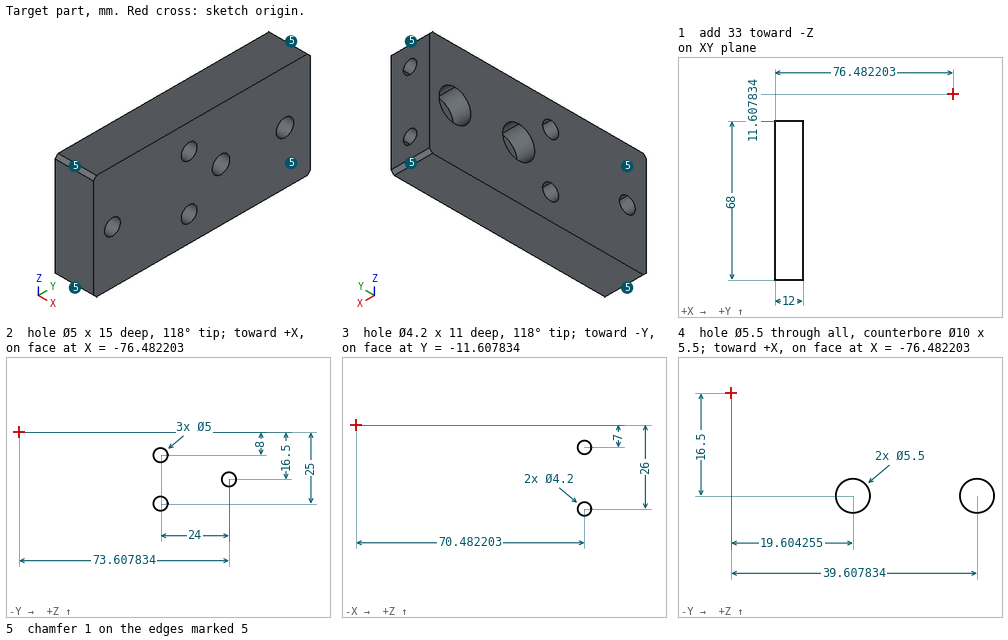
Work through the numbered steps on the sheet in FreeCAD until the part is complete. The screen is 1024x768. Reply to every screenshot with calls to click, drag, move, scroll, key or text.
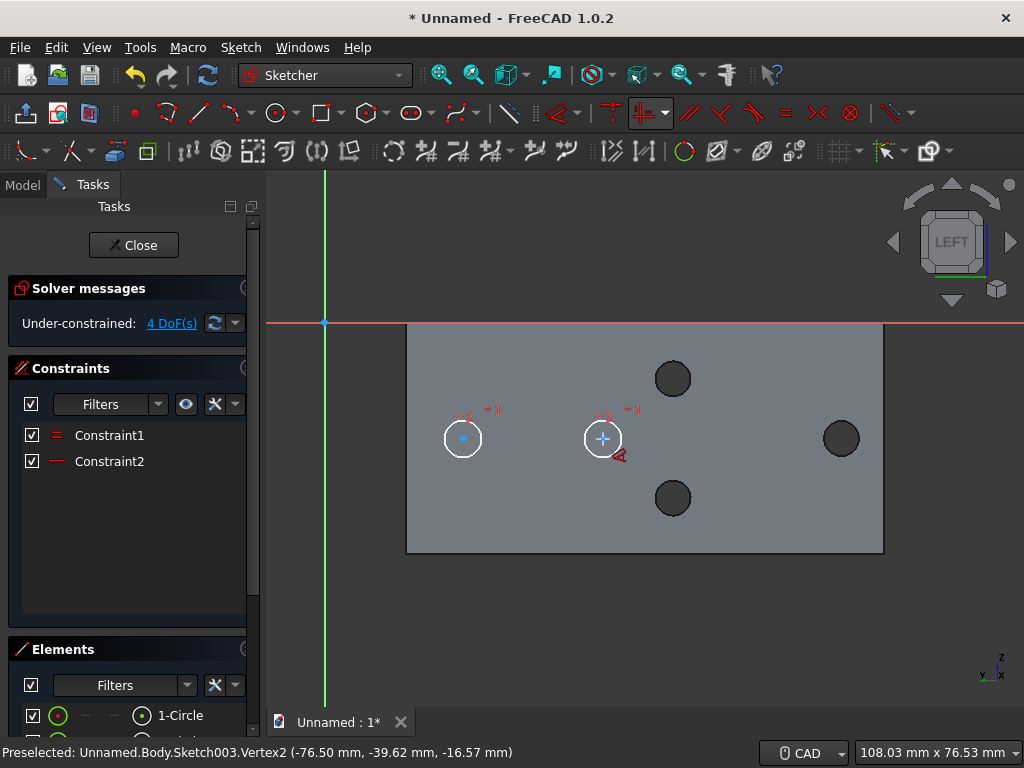
click(476, 426)
click(499, 403)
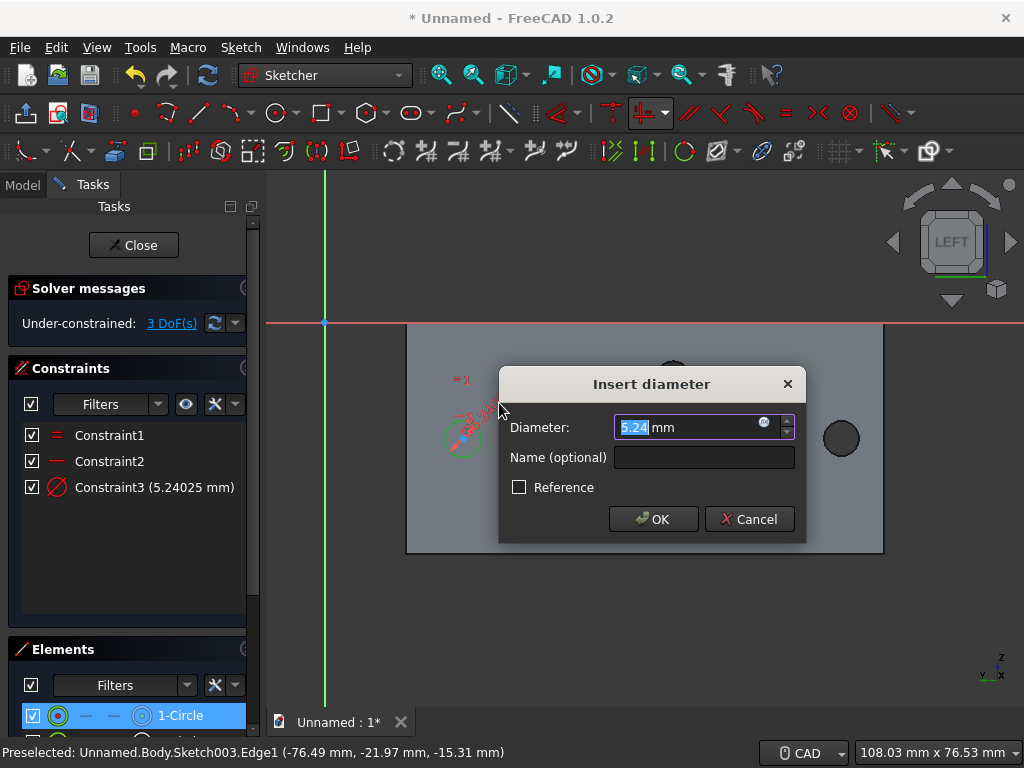
text(5.5)
key(Return)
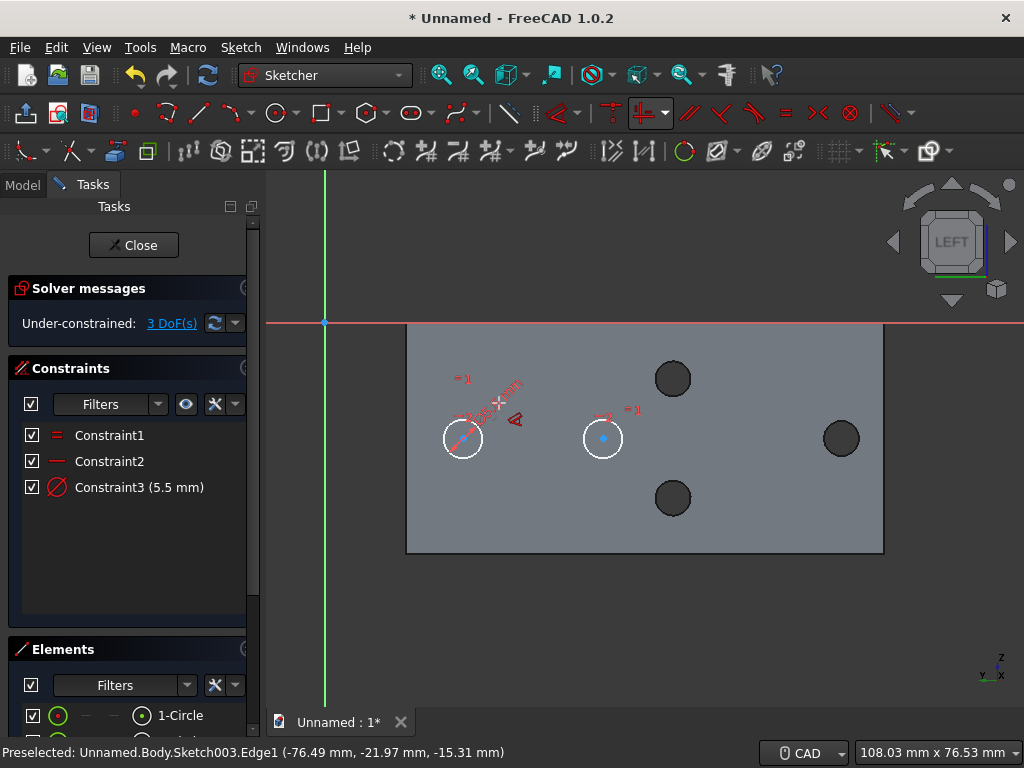
click(463, 439)
click(497, 381)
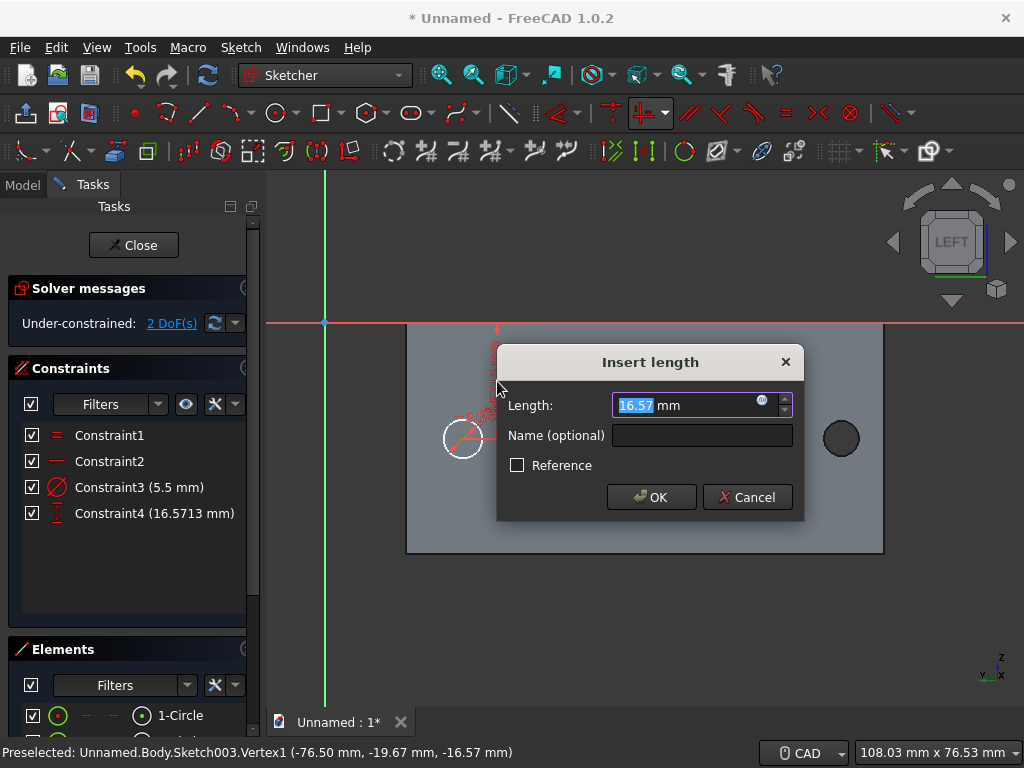
text(16.5)
key(Return)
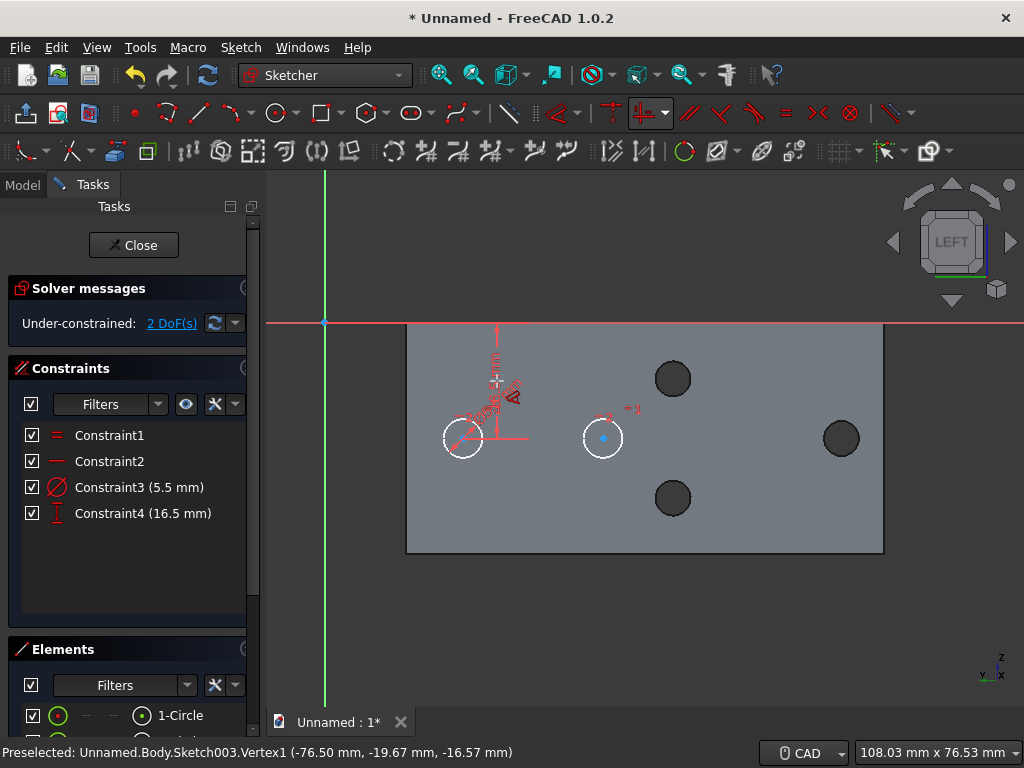
click(463, 438)
click(394, 289)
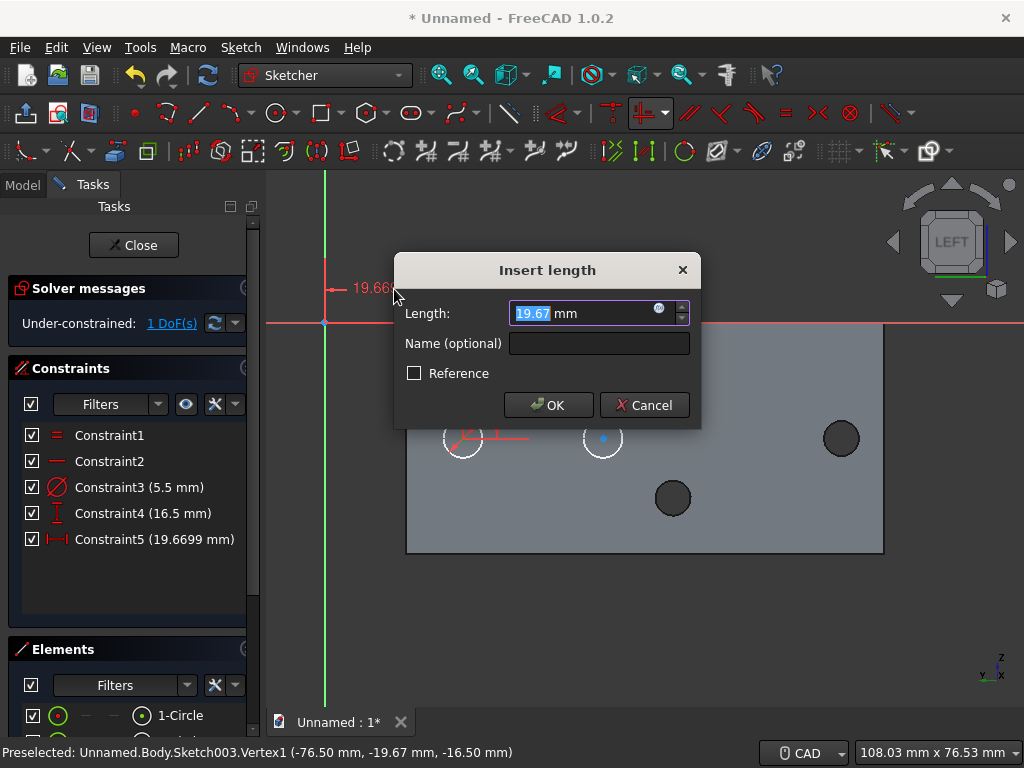
text(19.604255)
key(Return)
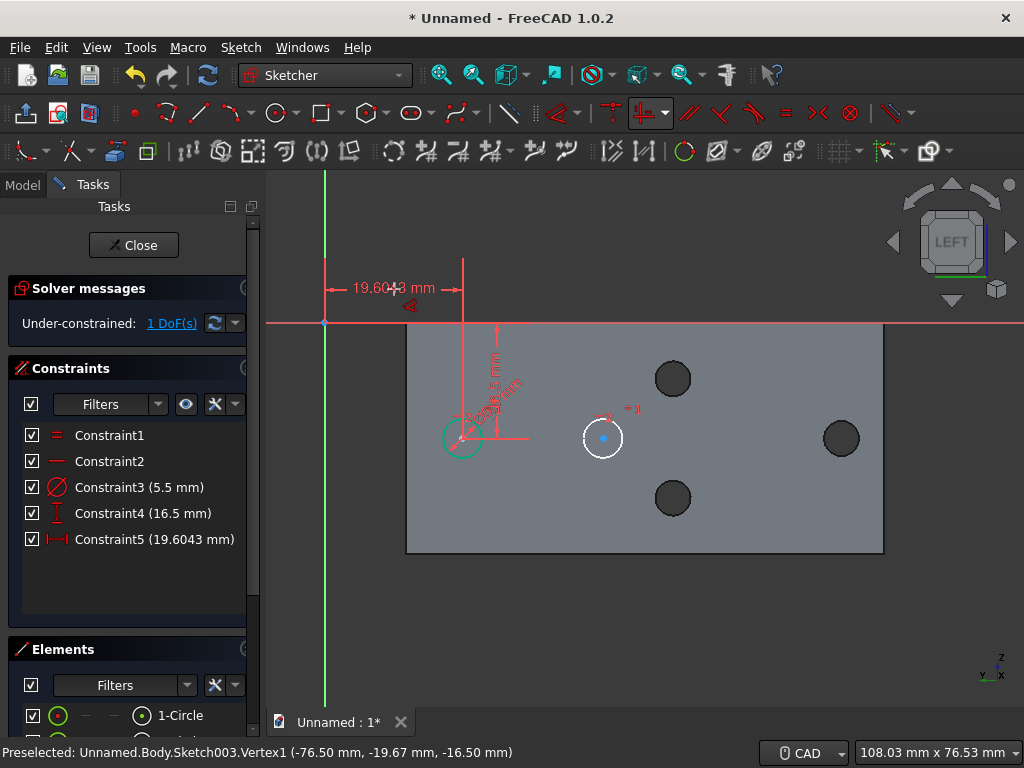
click(603, 438)
click(464, 289)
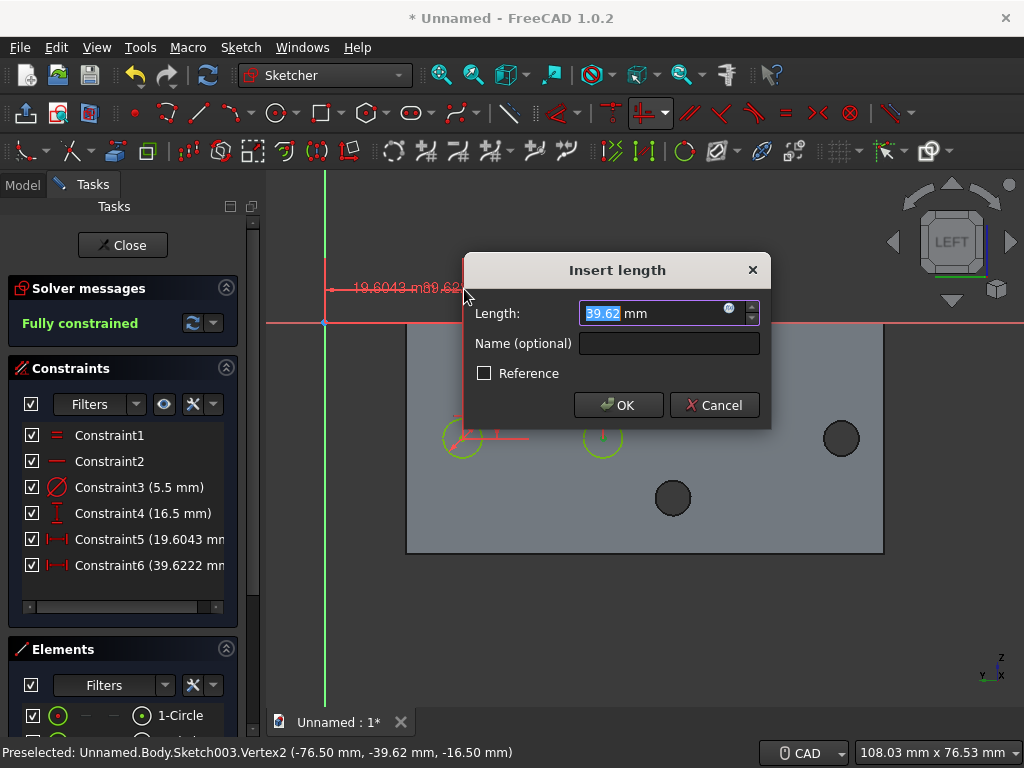
text(39.607834)
key(Return)
key(Escape)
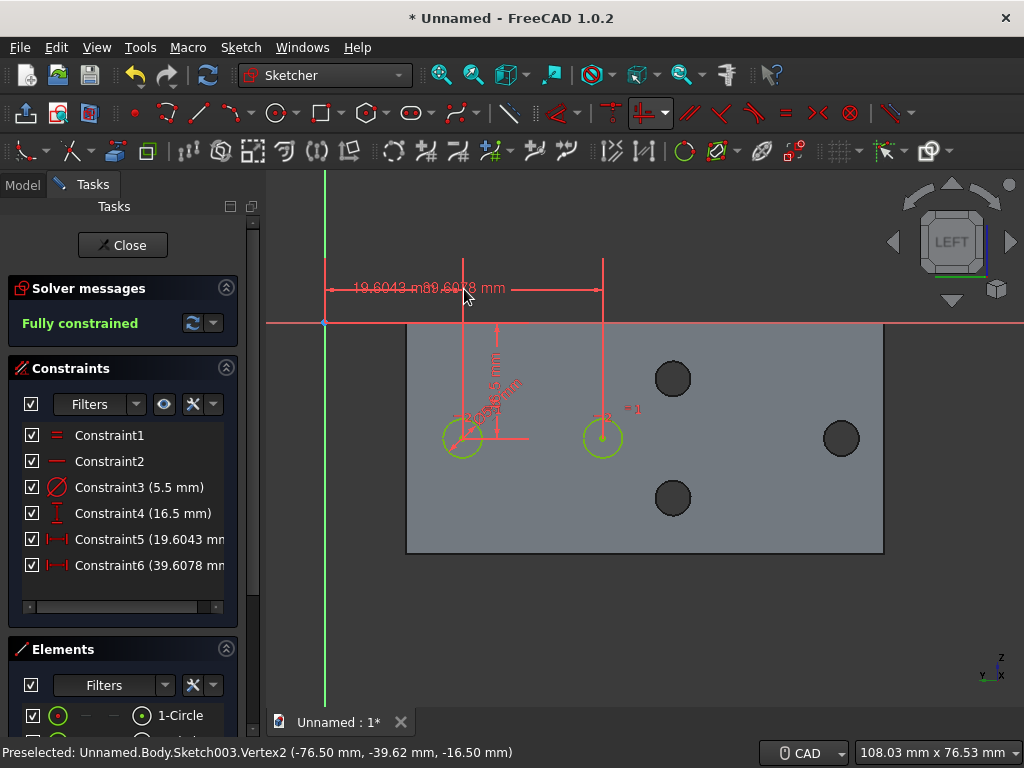
click(123, 245)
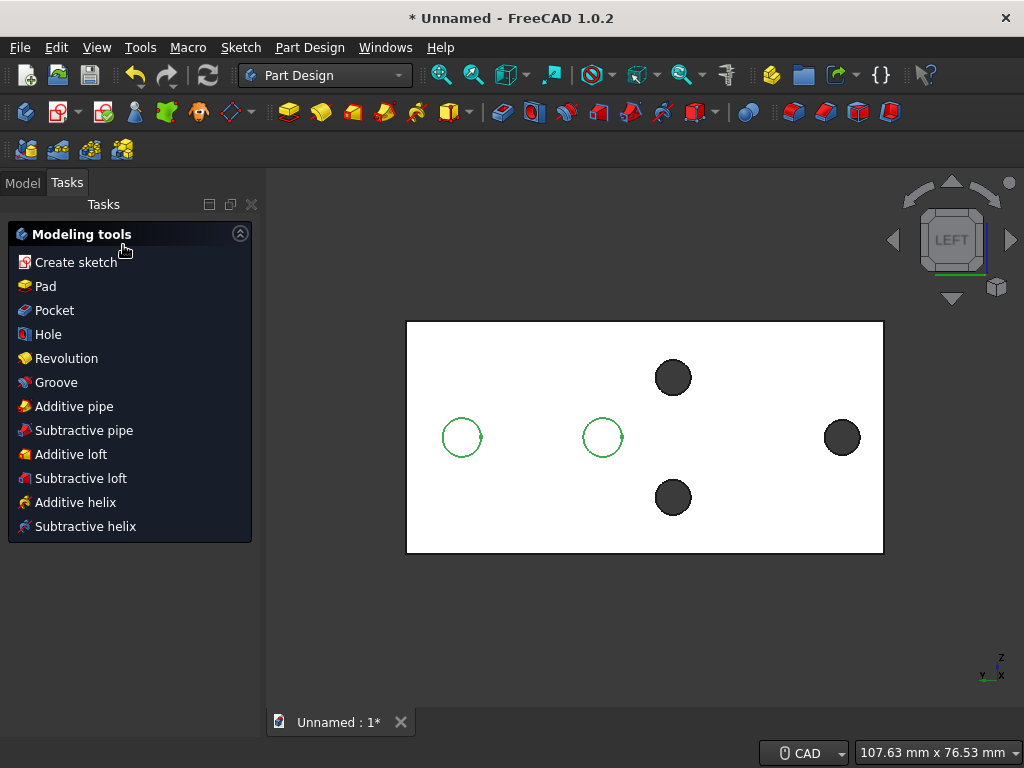
click(536, 112)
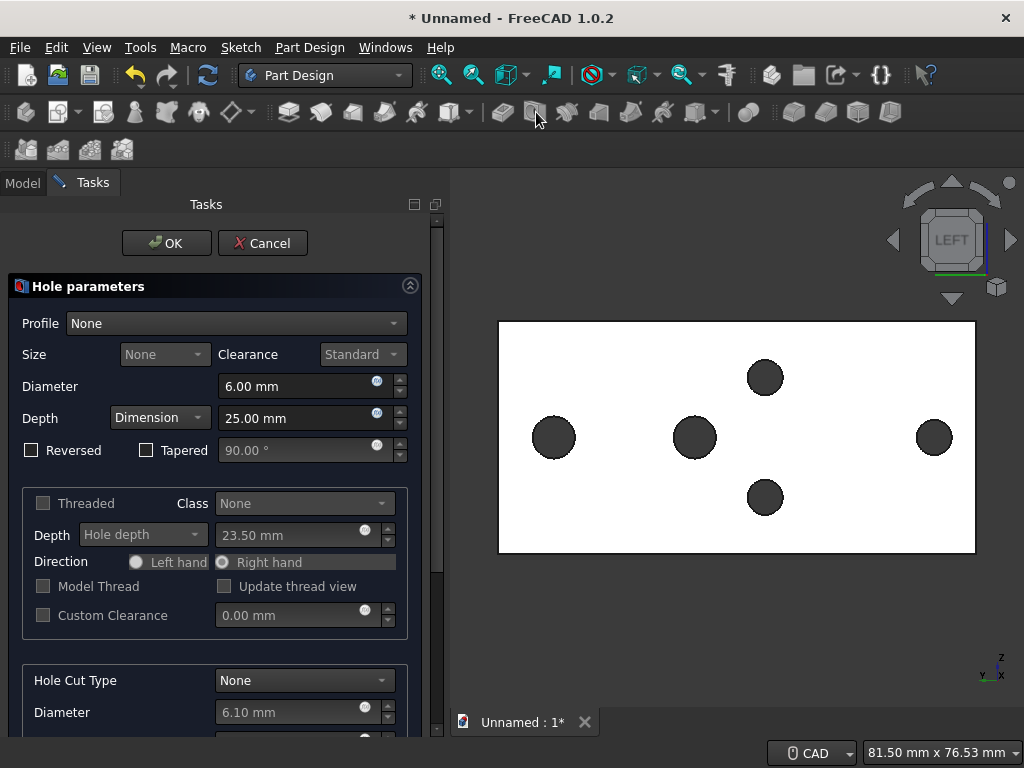
triple_click(305, 386)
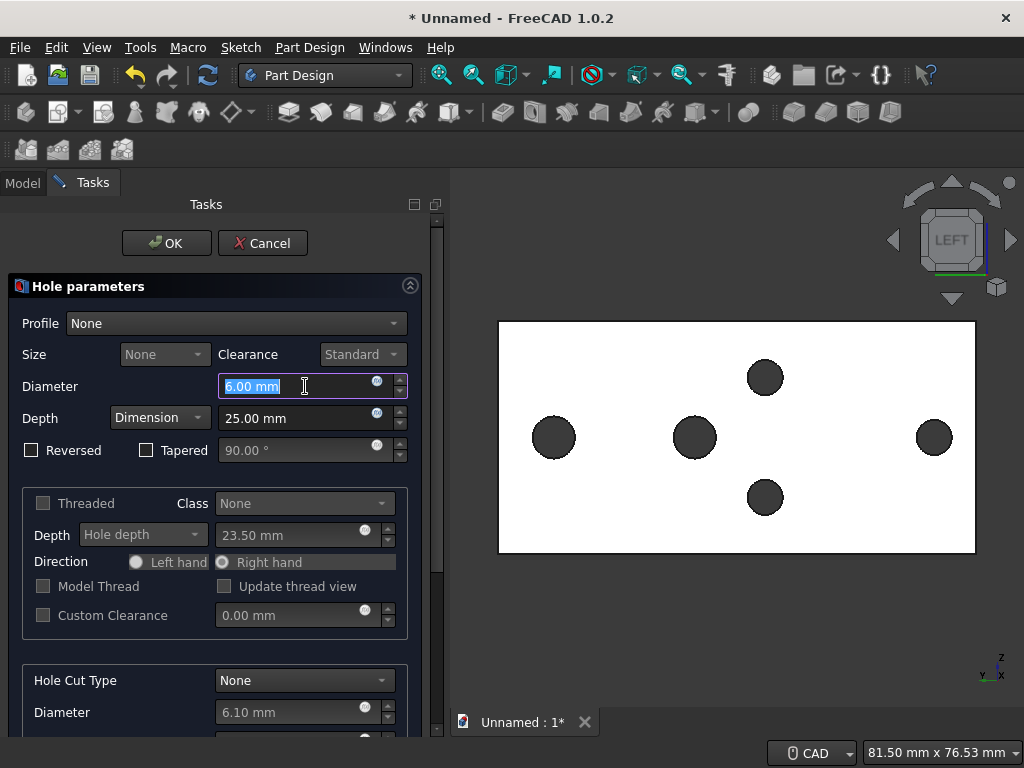
text(5.5)
key(Tab)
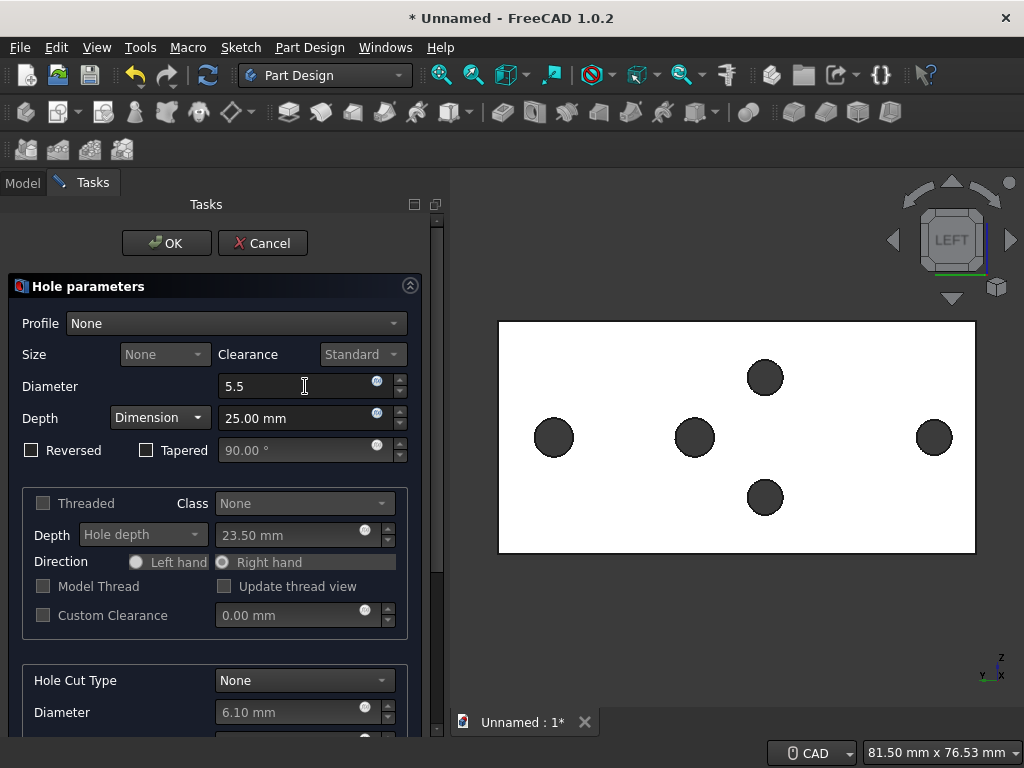
click(161, 418)